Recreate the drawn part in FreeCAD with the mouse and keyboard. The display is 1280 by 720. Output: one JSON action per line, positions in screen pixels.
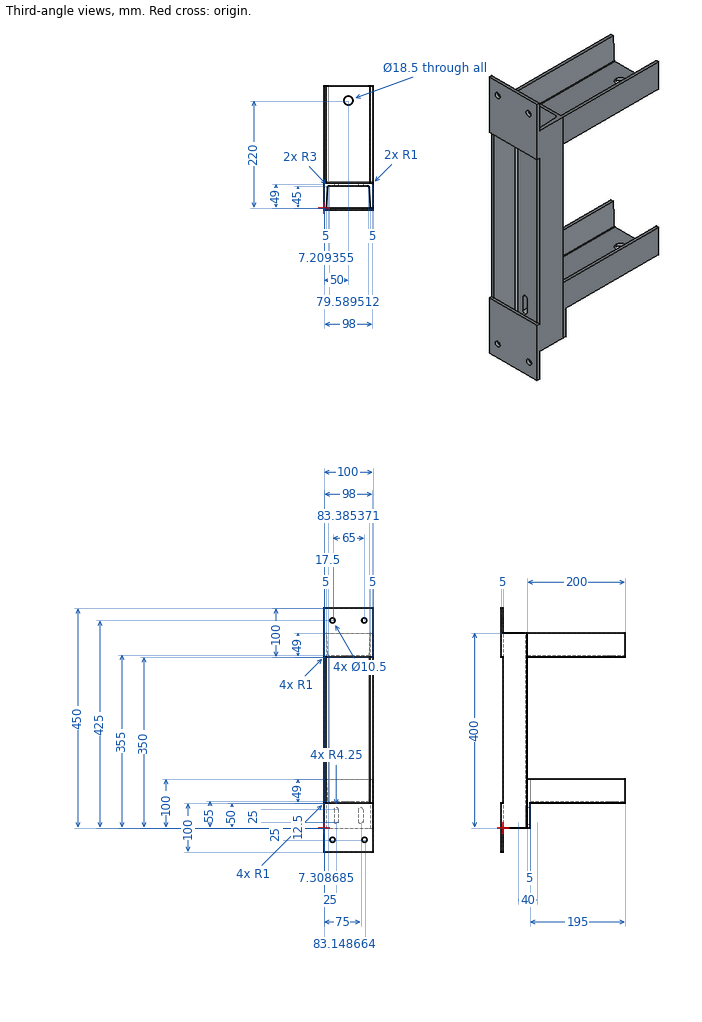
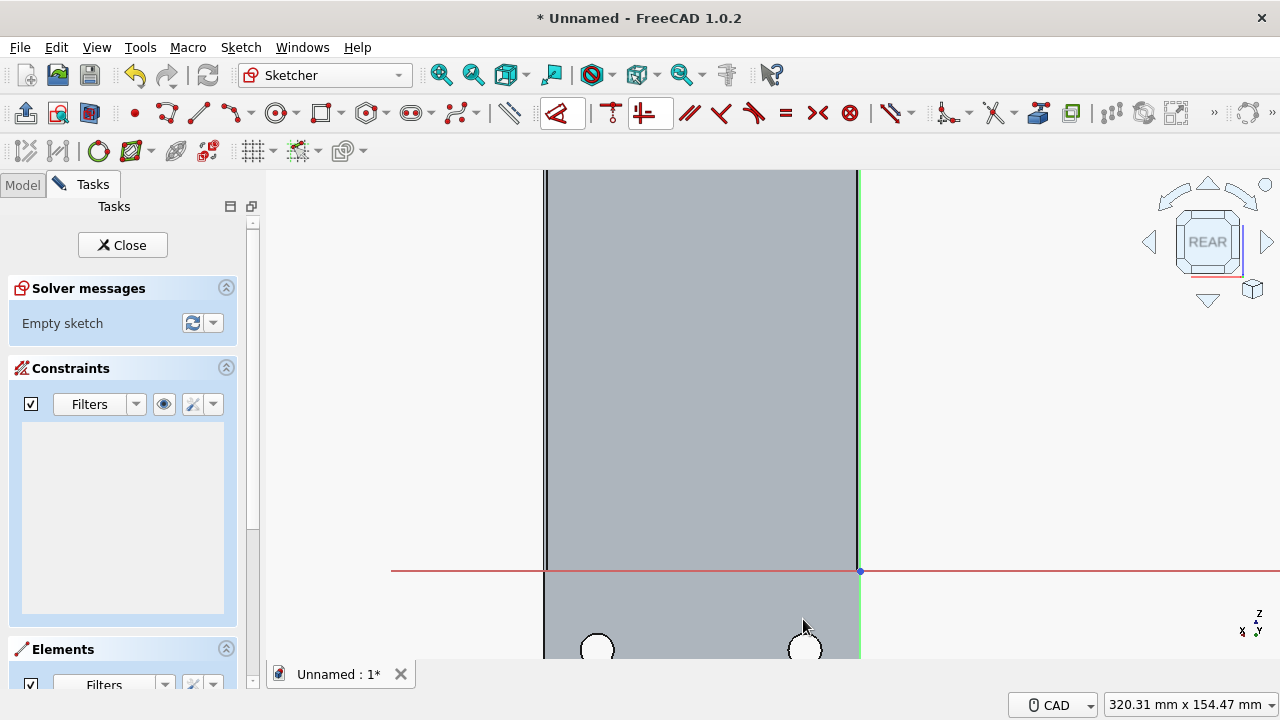
{"action": "left_click", "coordinate": [322, 114]}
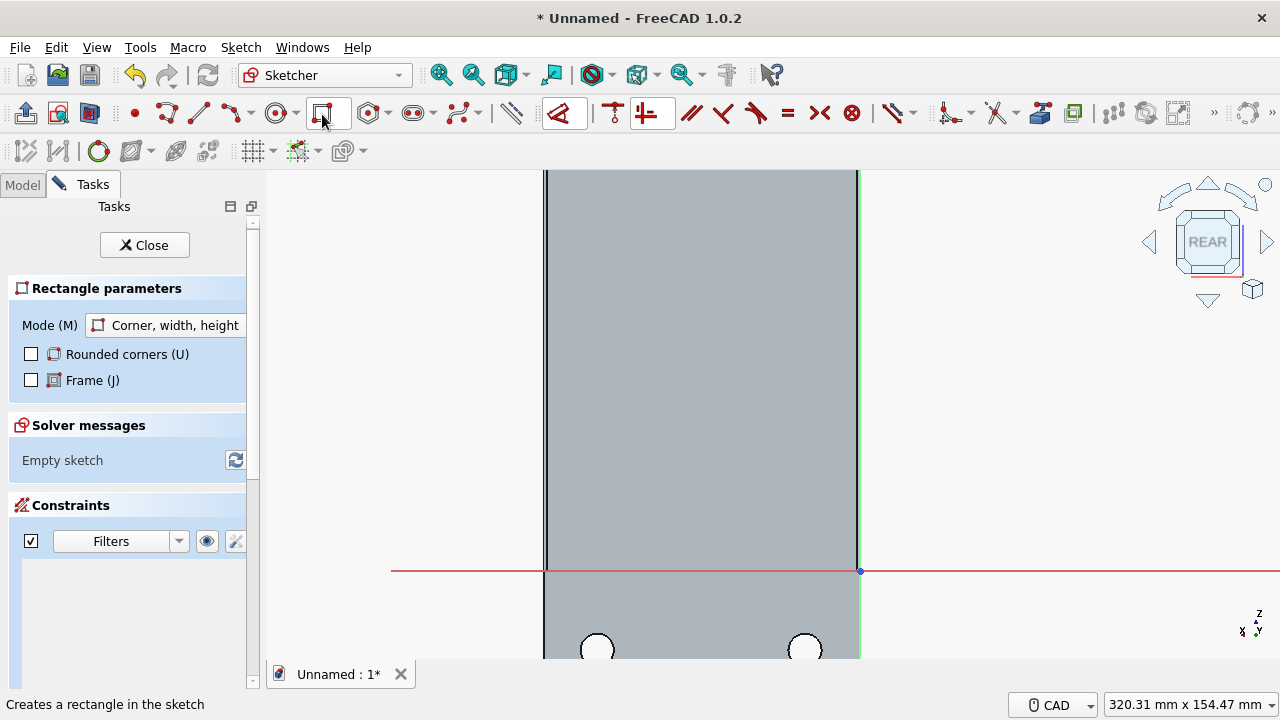
{"action": "left_click", "coordinate": [860, 571]}
{"action": "left_click", "coordinate": [544, 254]}
{"action": "key", "text": "Escape"}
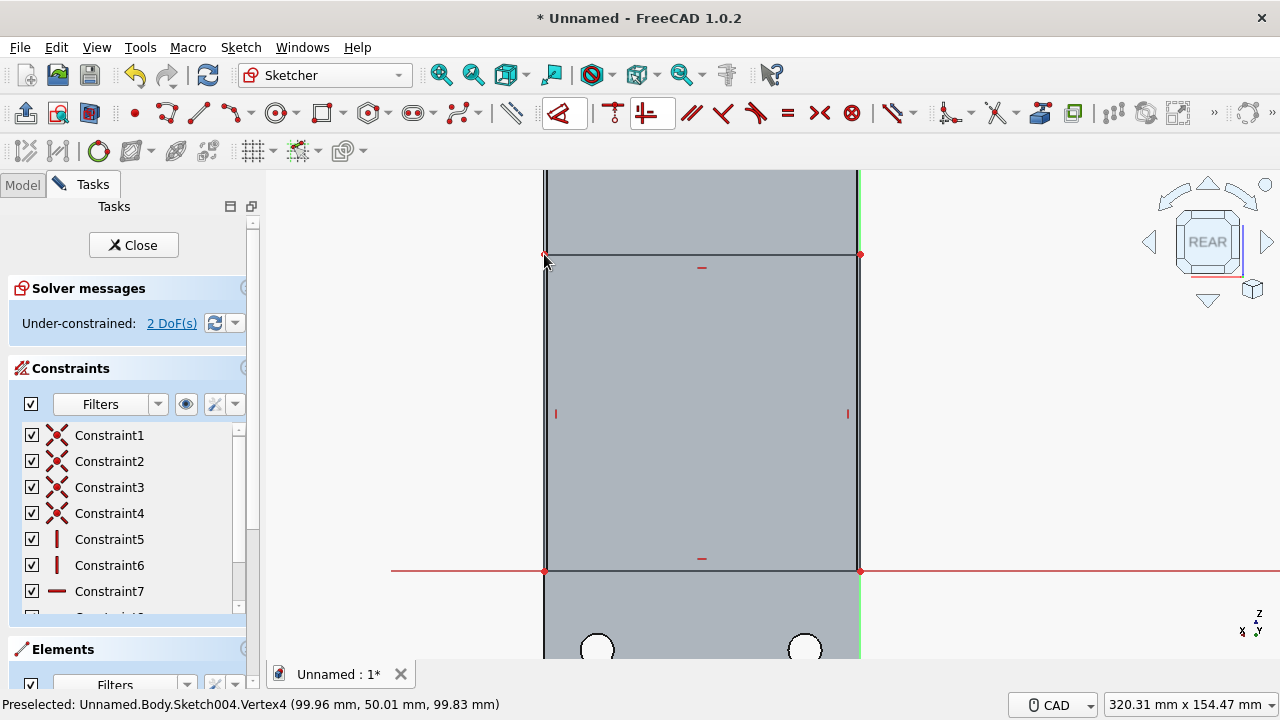
{"action": "left_click", "coordinate": [860, 476]}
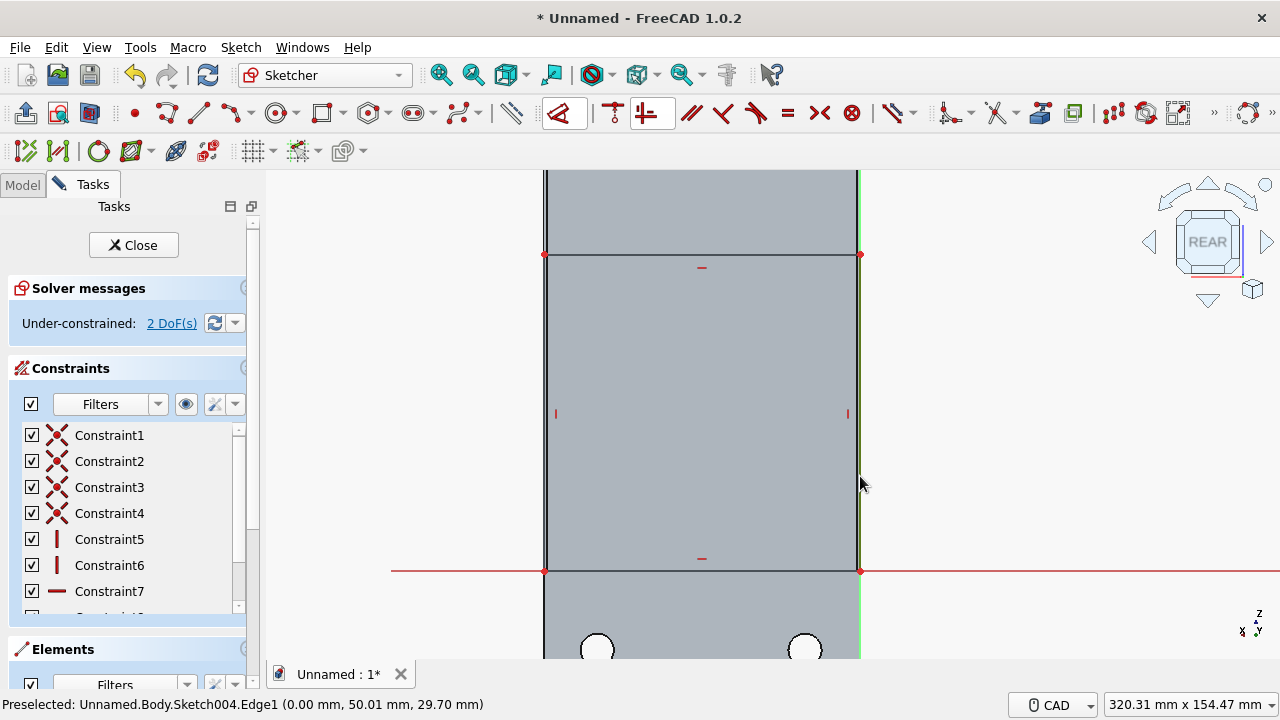
{"action": "left_click", "coordinate": [582, 114]}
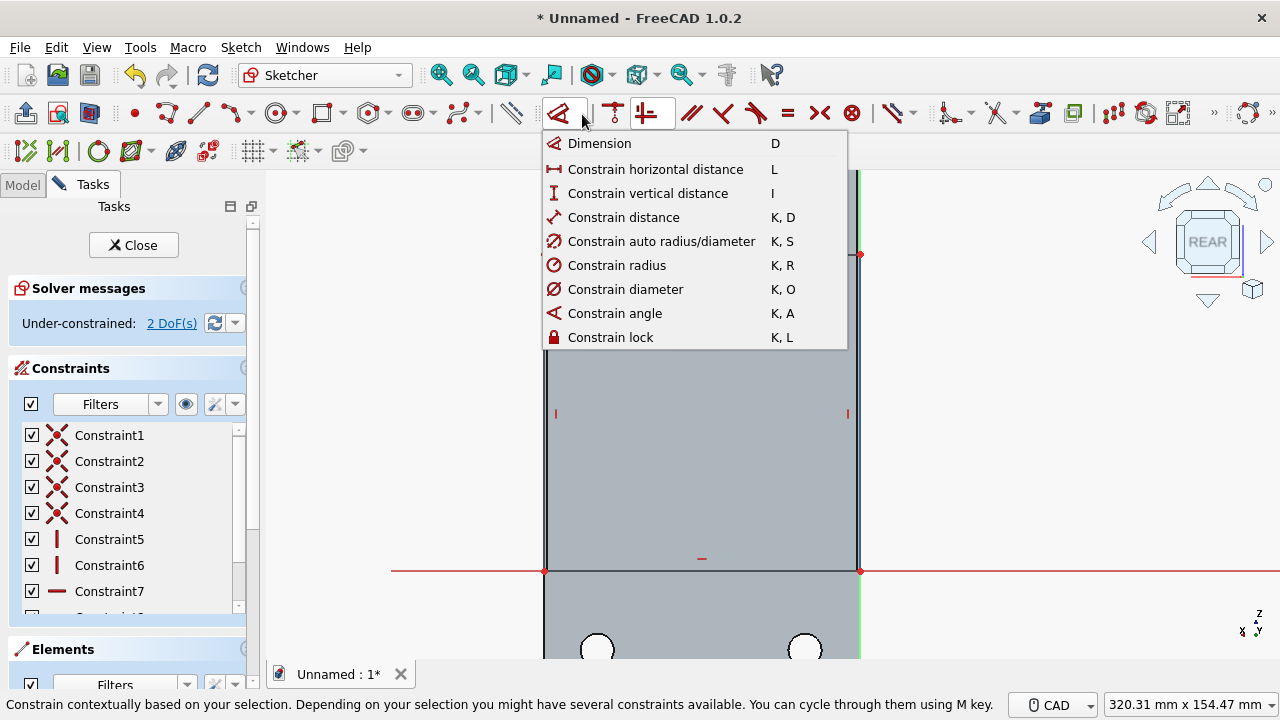
{"action": "left_click", "coordinate": [695, 193]}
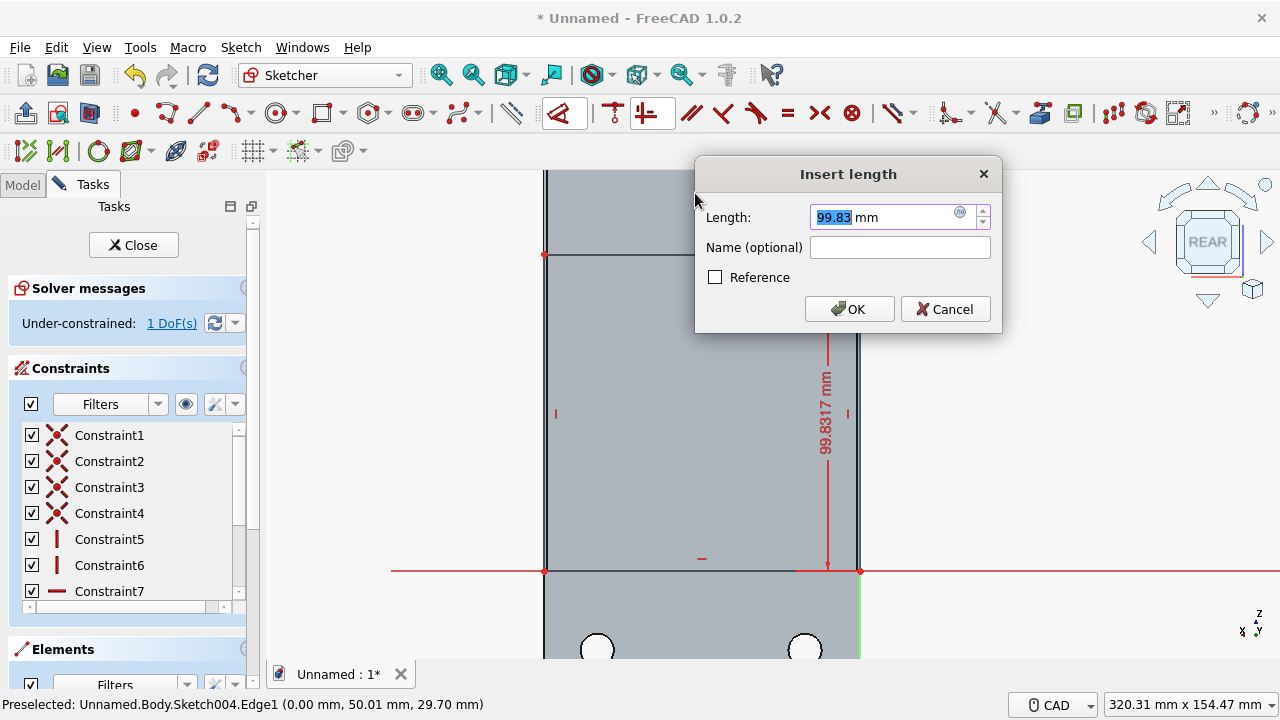
{"action": "type", "text": "100"}
{"action": "key", "text": "Return"}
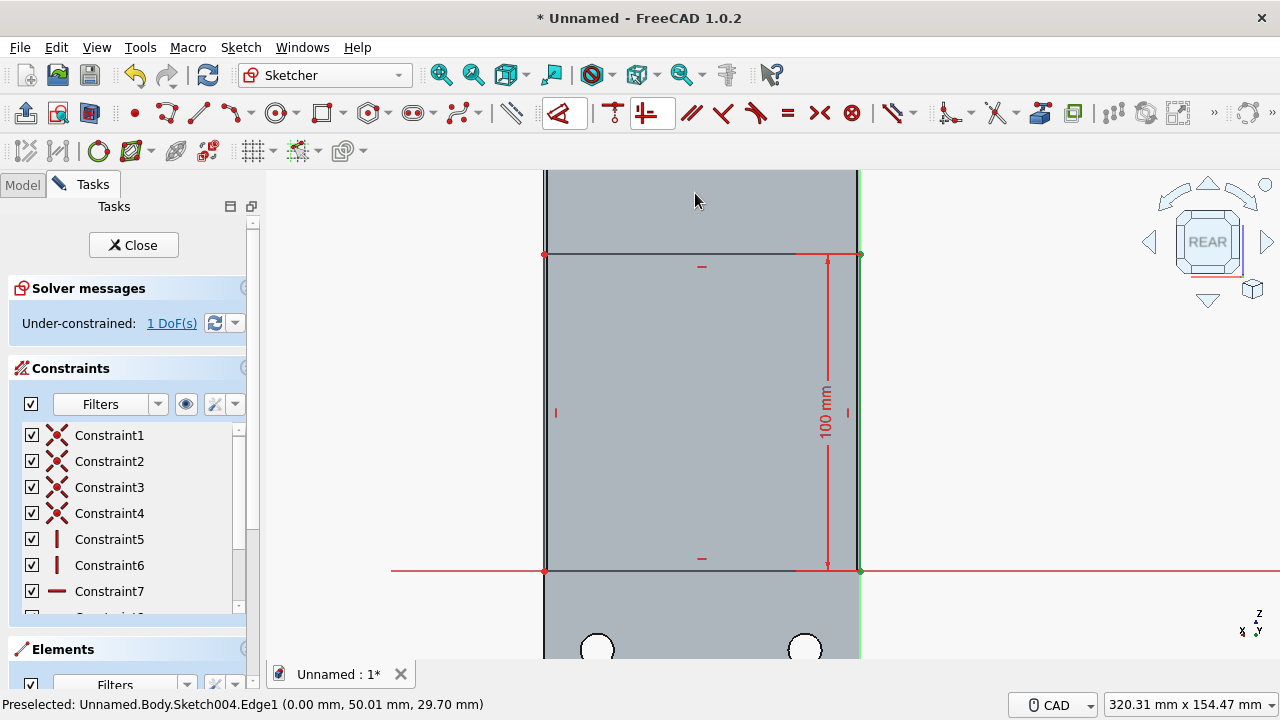
{"action": "left_click", "coordinate": [766, 254]}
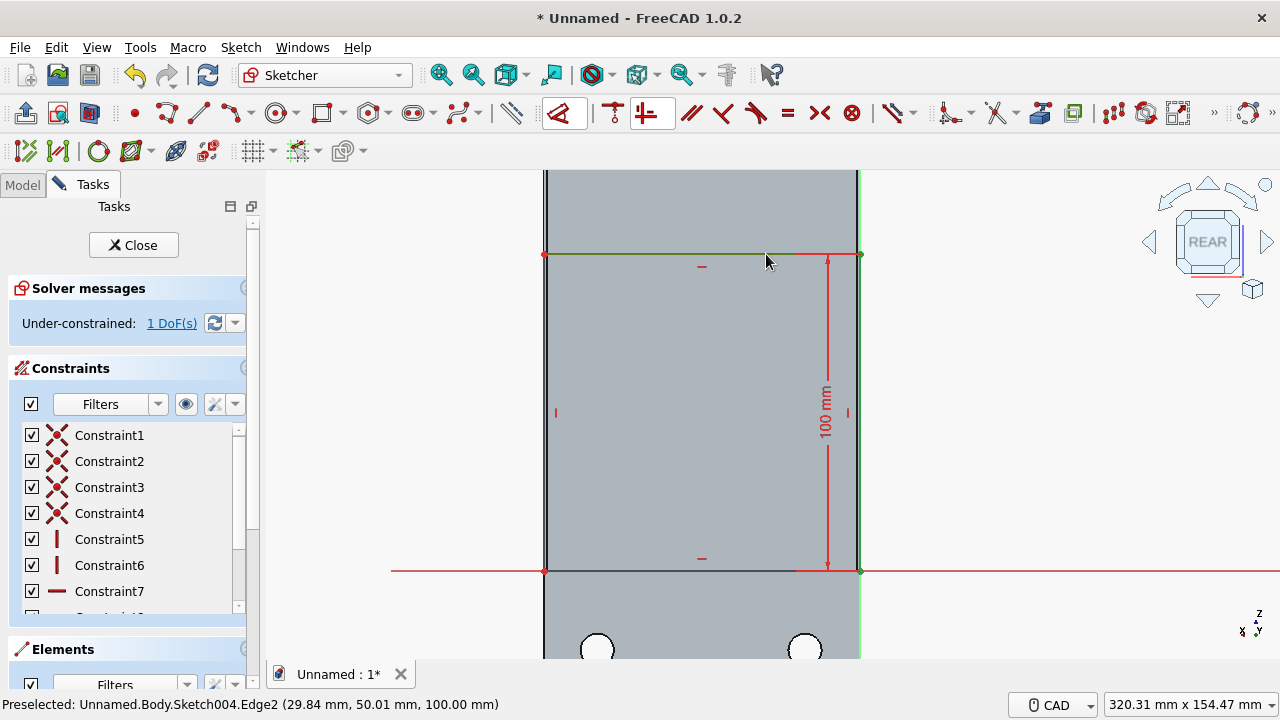
{"action": "left_click", "coordinate": [582, 114]}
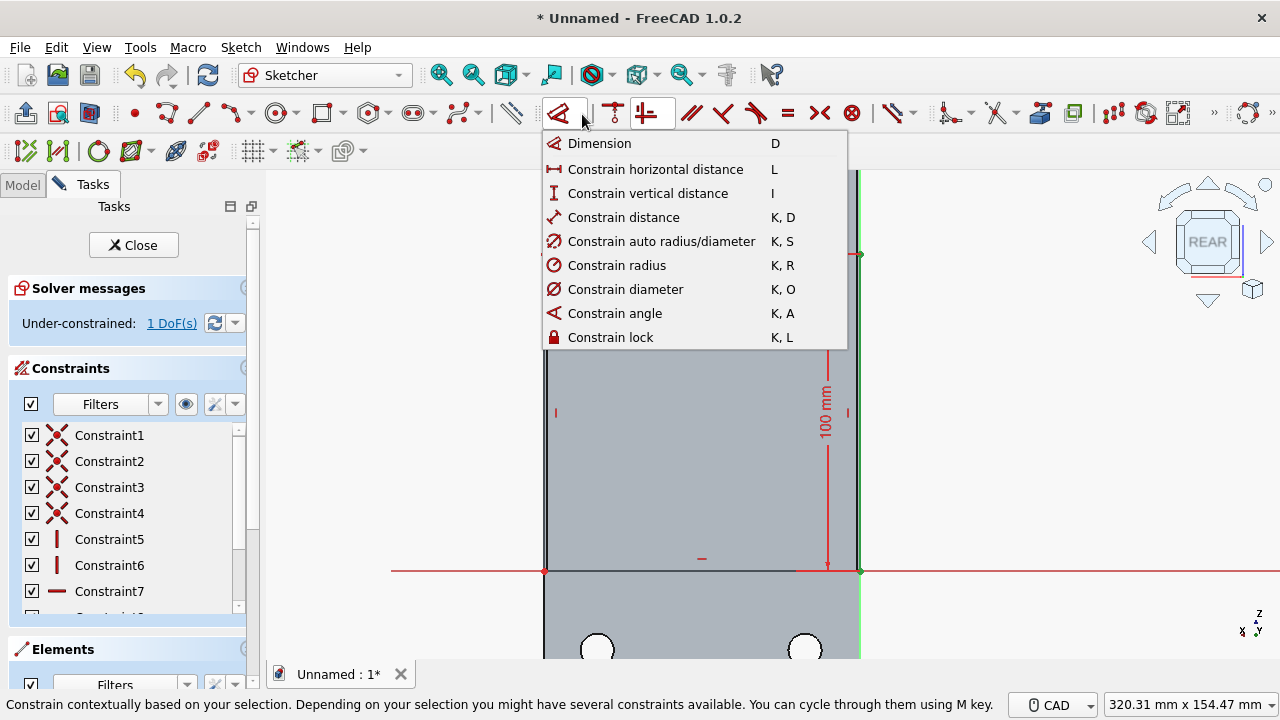
{"action": "left_click", "coordinate": [695, 169]}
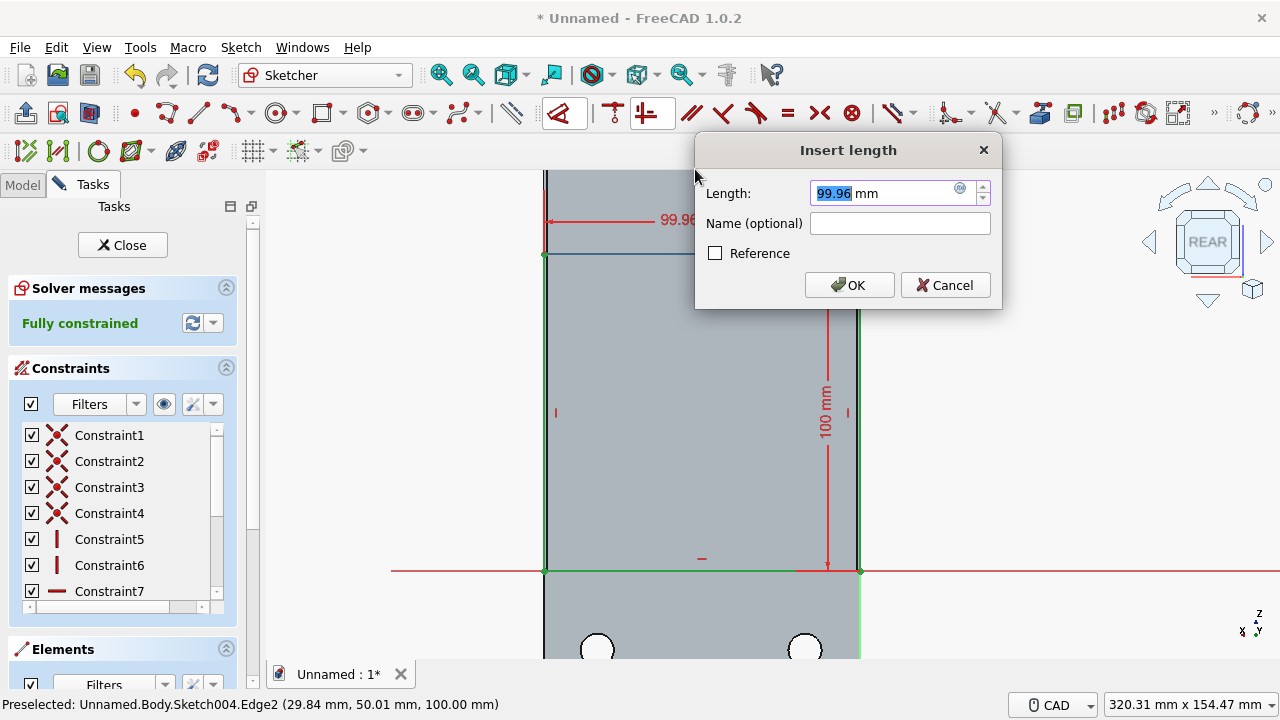
{"action": "type", "text": "100"}
{"action": "key", "text": "Return"}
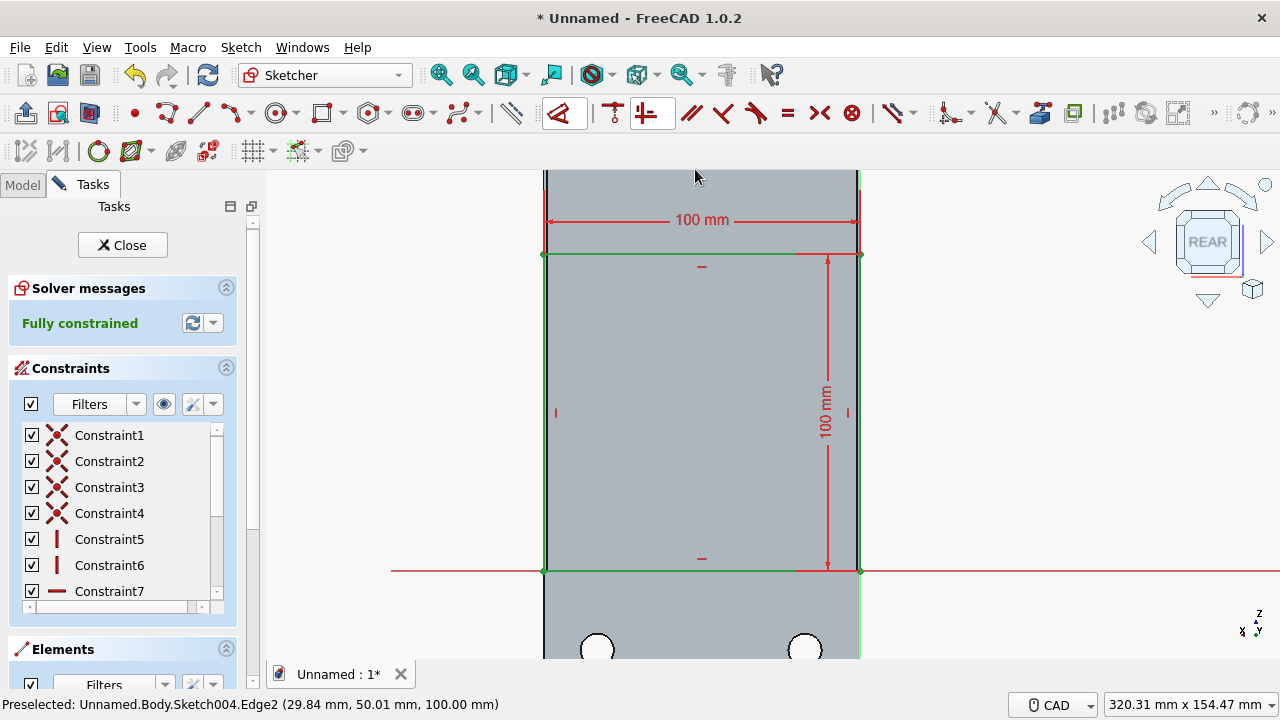
{"action": "left_click", "coordinate": [123, 245]}